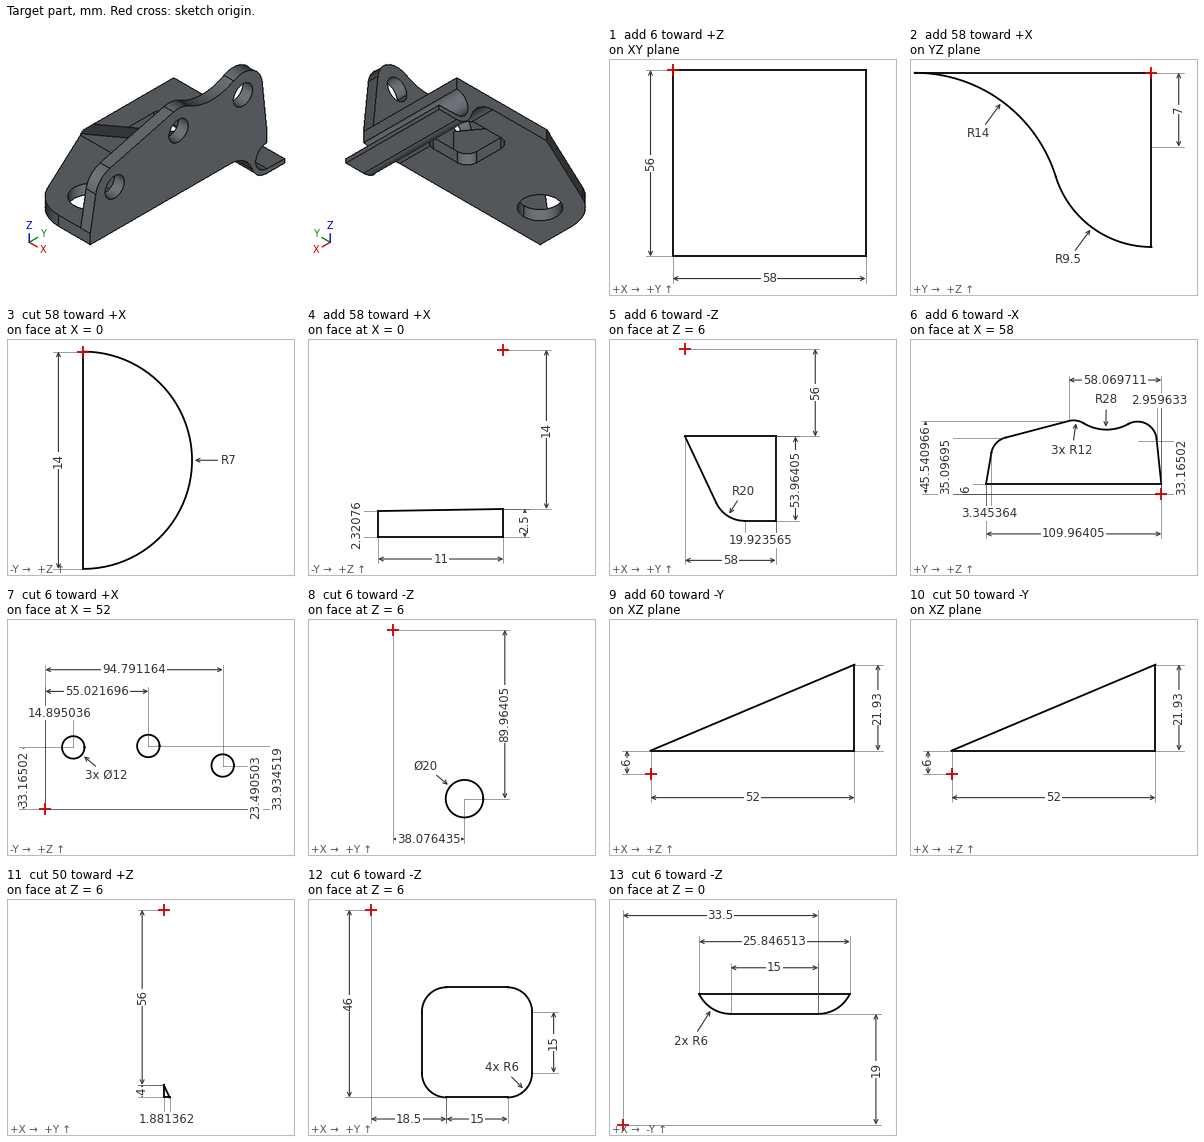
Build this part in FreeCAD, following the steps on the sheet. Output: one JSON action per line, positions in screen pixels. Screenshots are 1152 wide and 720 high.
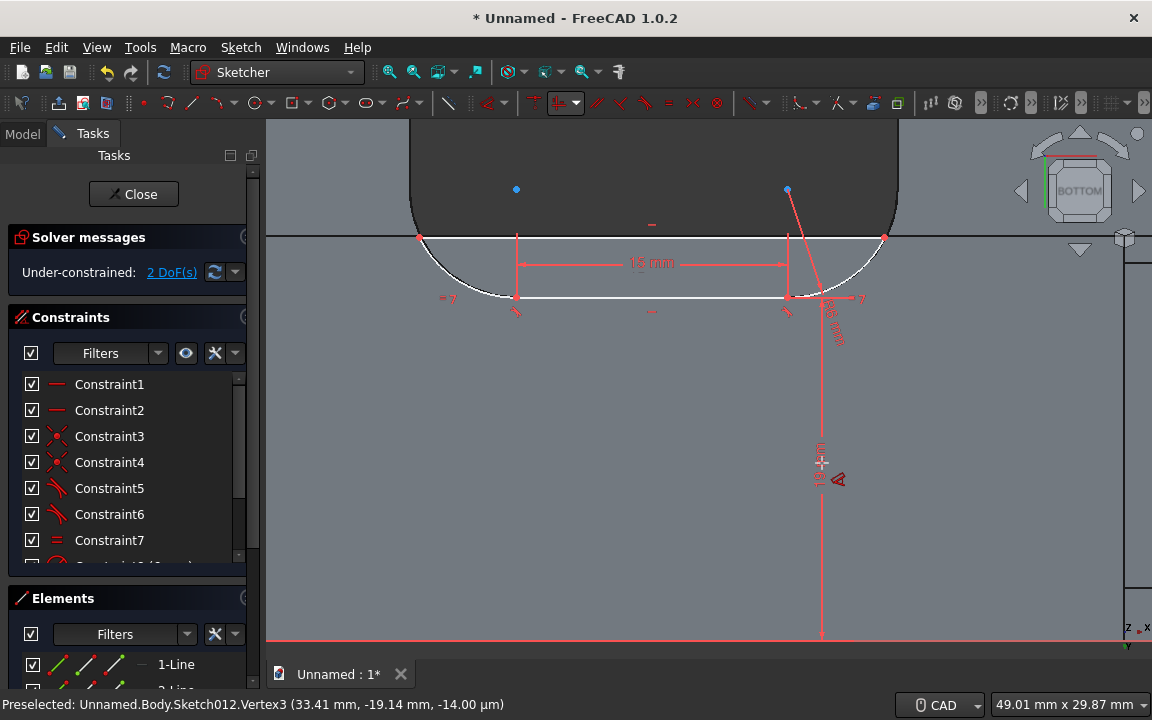
{"action": "left_click", "coordinate": [788, 298]}
{"action": "left_click", "coordinate": [541, 264]}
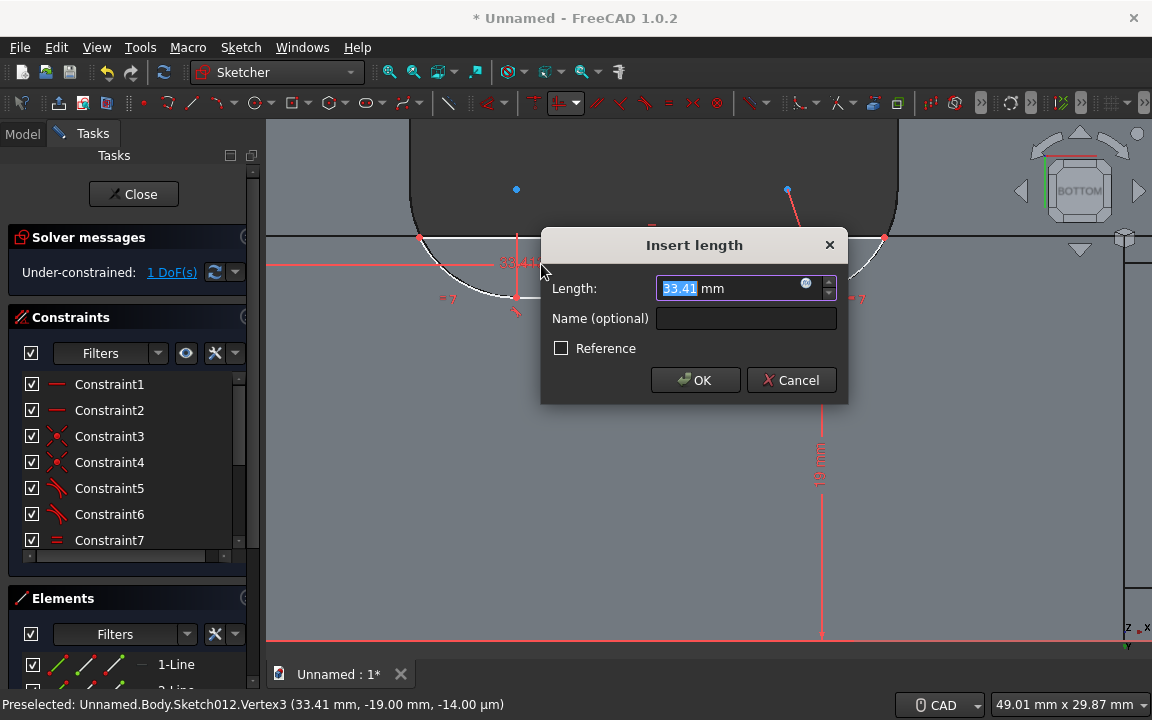
{"action": "type", "text": "33.5"}
{"action": "key", "text": "Return"}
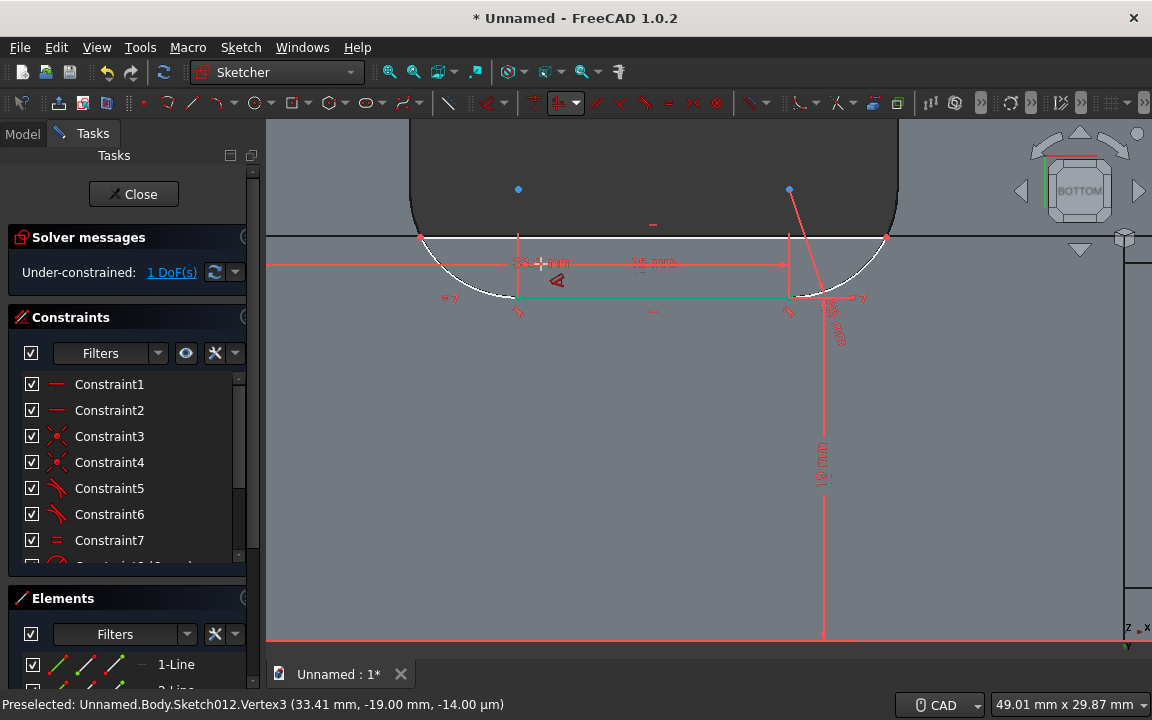
{"action": "left_click", "coordinate": [561, 238]}
{"action": "left_click", "coordinate": [654, 204]}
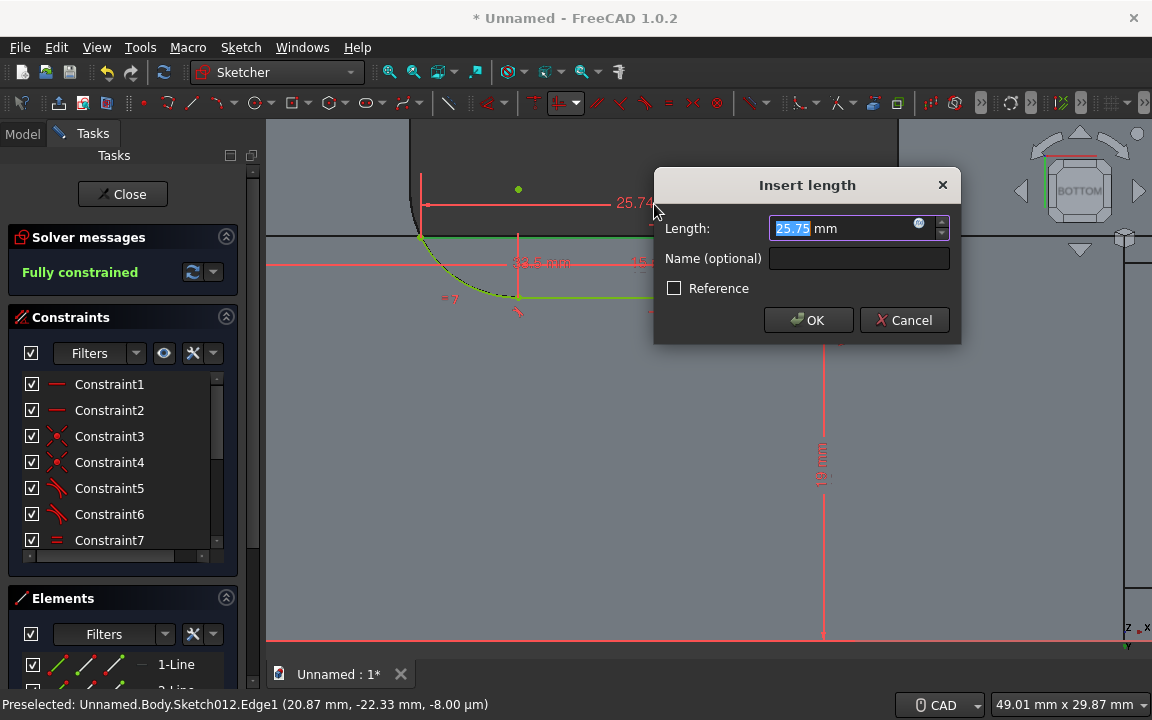
{"action": "type", "text": "25.846513"}
{"action": "key", "text": "Return"}
{"action": "key", "text": "Escape"}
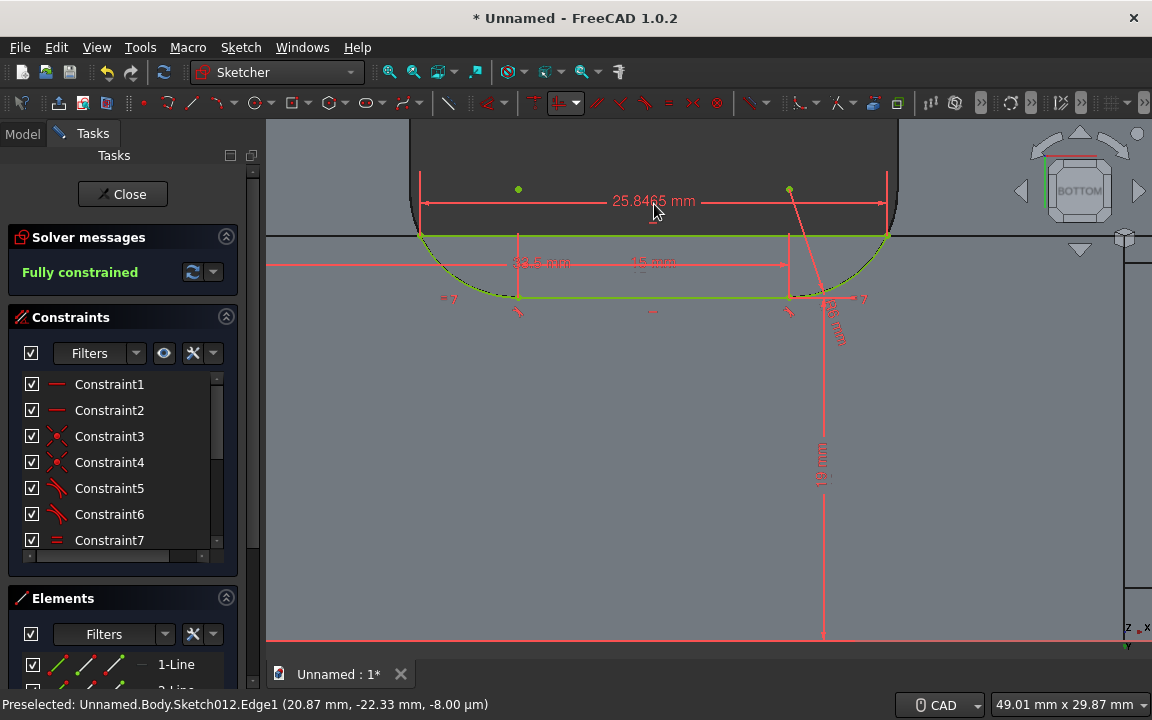
{"action": "left_click", "coordinate": [123, 194]}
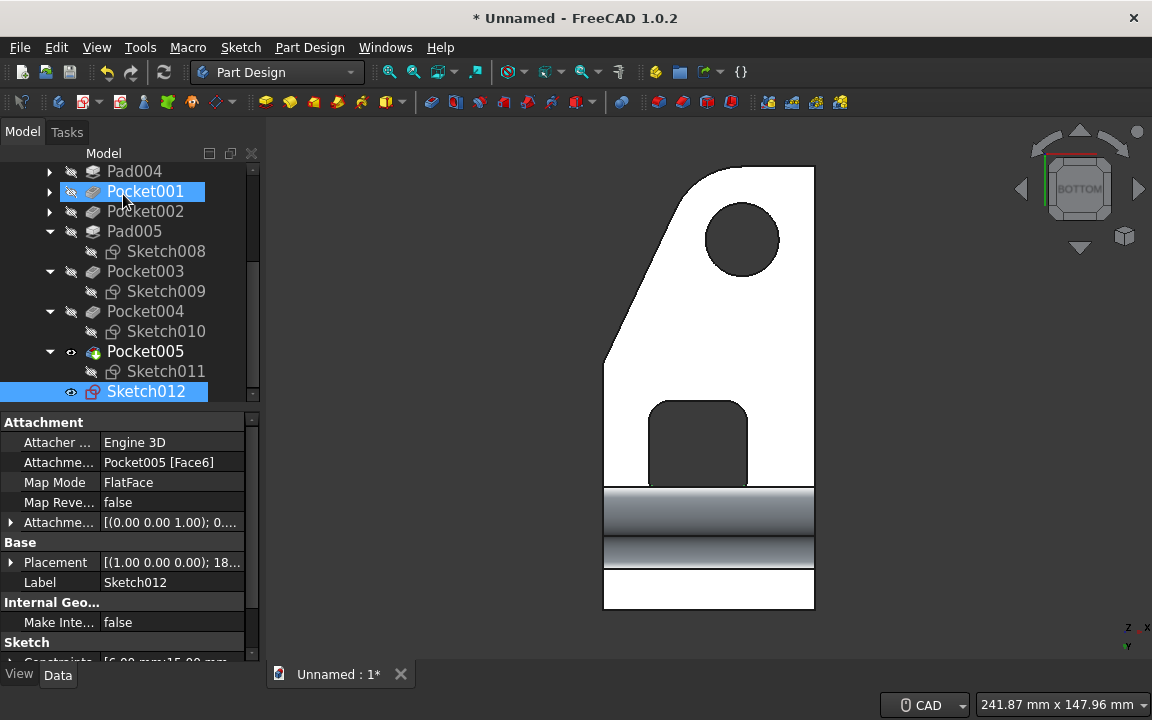
{"action": "left_click", "coordinate": [432, 102]}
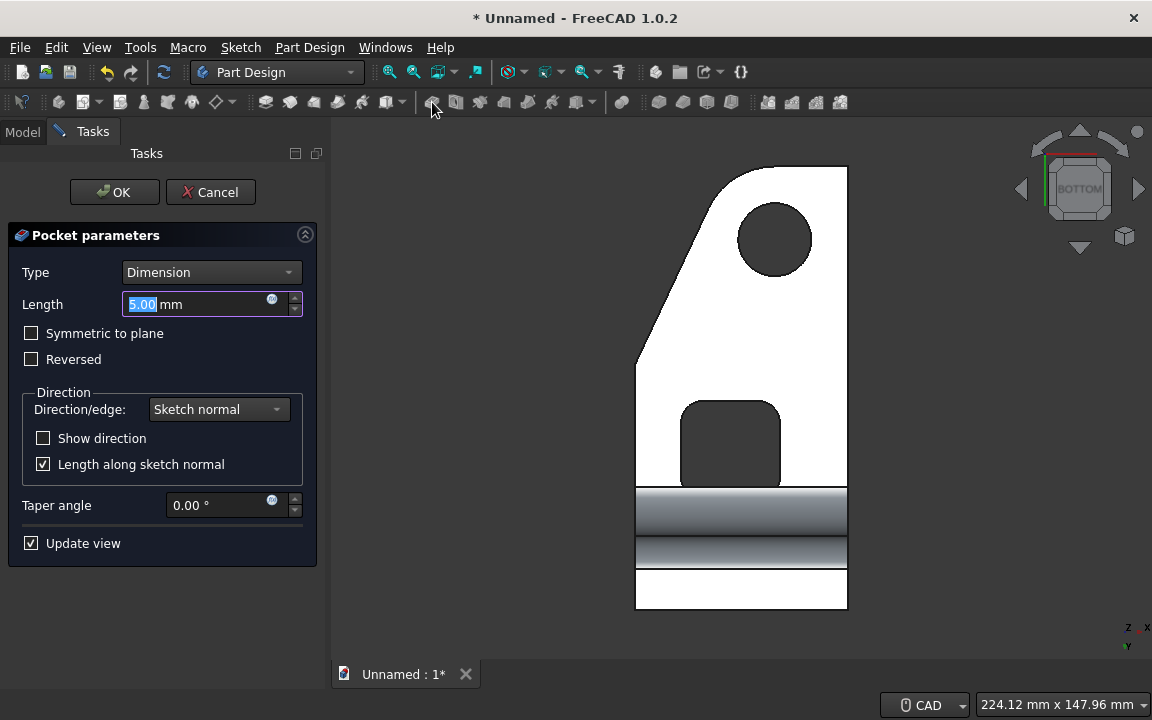
{"action": "type", "text": "6"}
{"action": "key", "text": "Tab"}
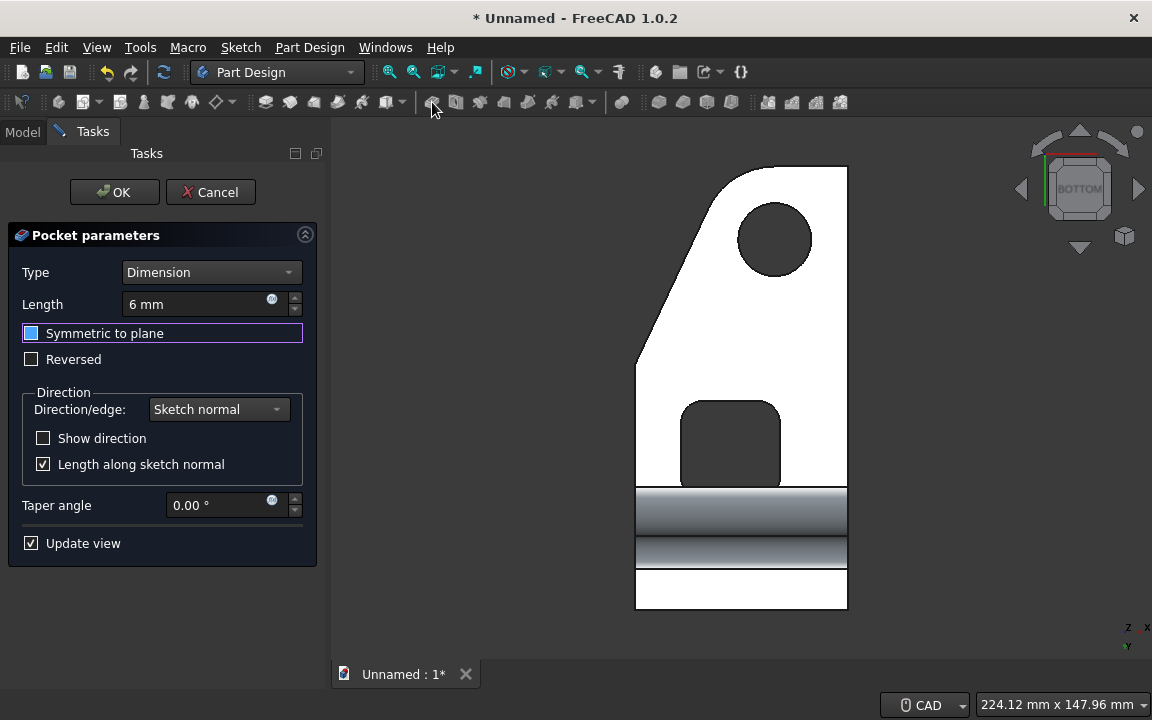
{"action": "left_click", "coordinate": [30, 359]}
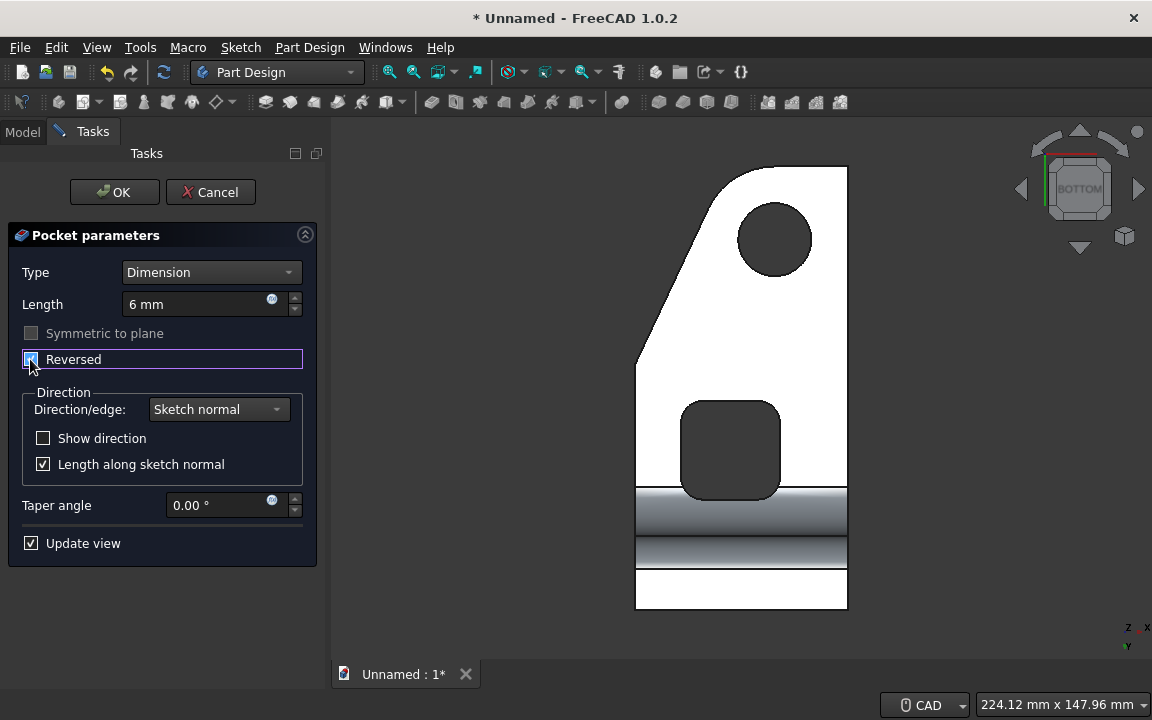
{"action": "left_click", "coordinate": [115, 192]}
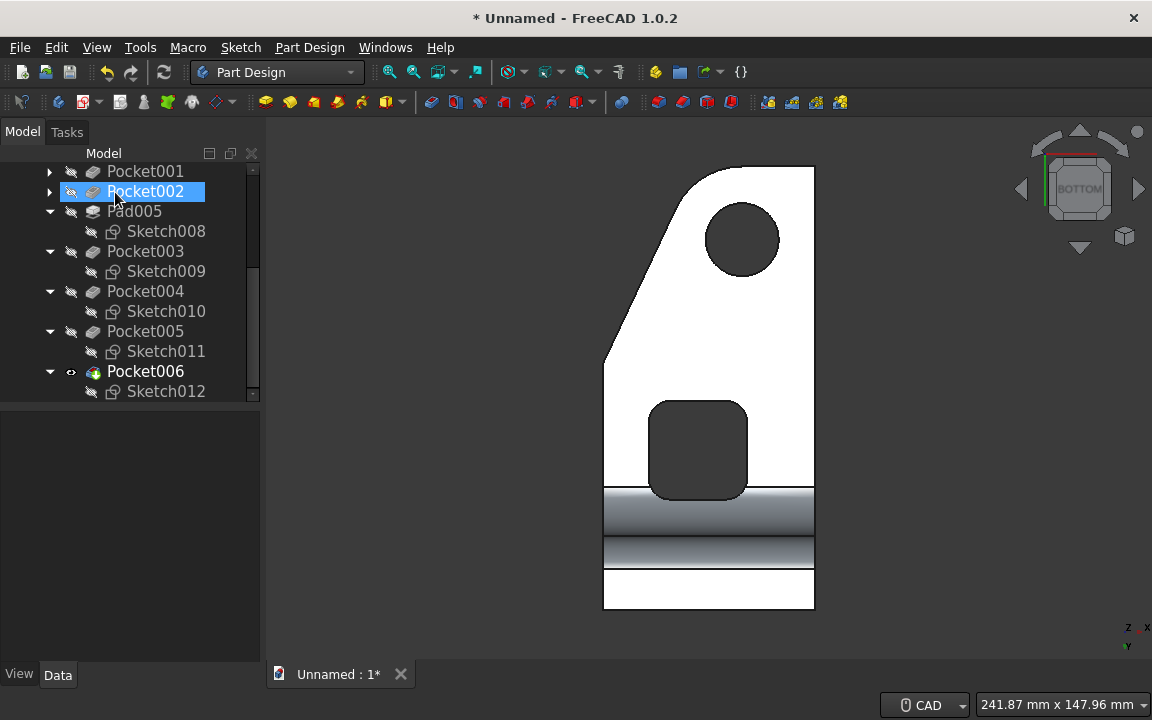
{"action": "key", "text": "0"}